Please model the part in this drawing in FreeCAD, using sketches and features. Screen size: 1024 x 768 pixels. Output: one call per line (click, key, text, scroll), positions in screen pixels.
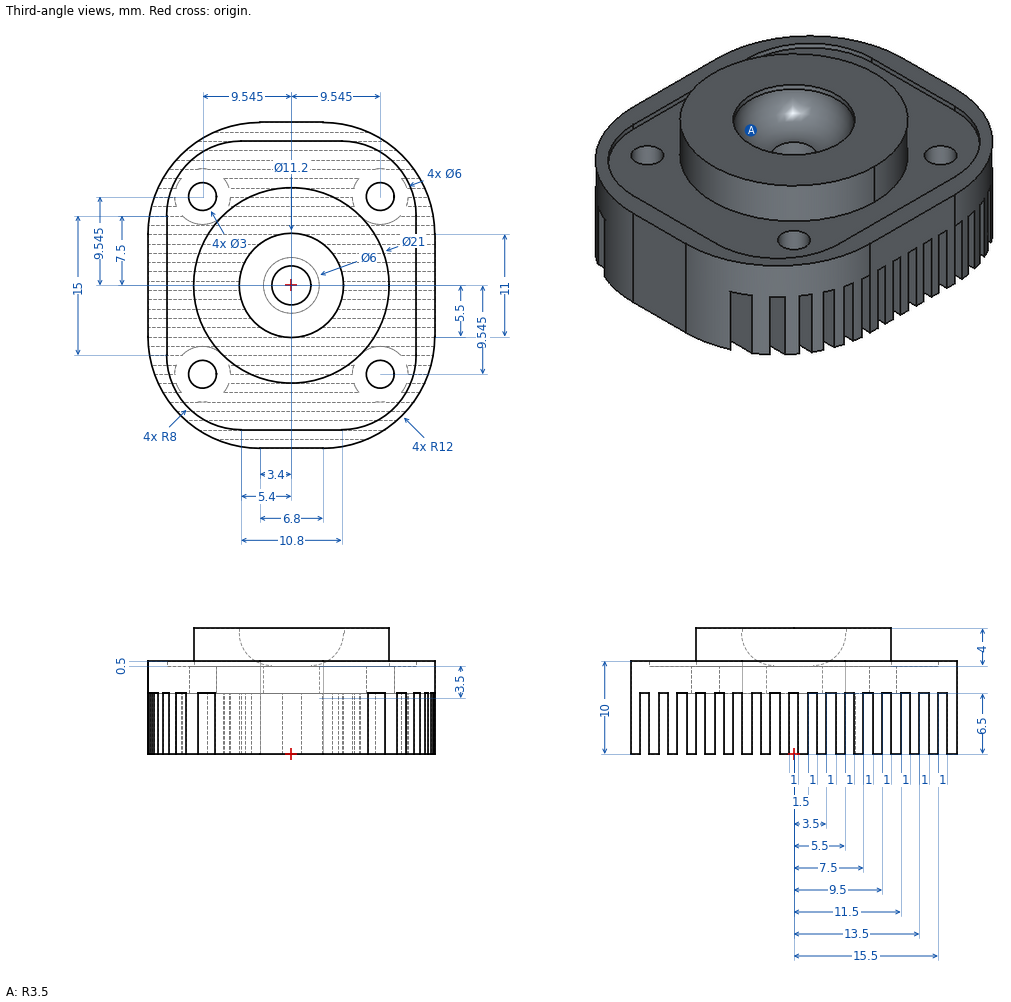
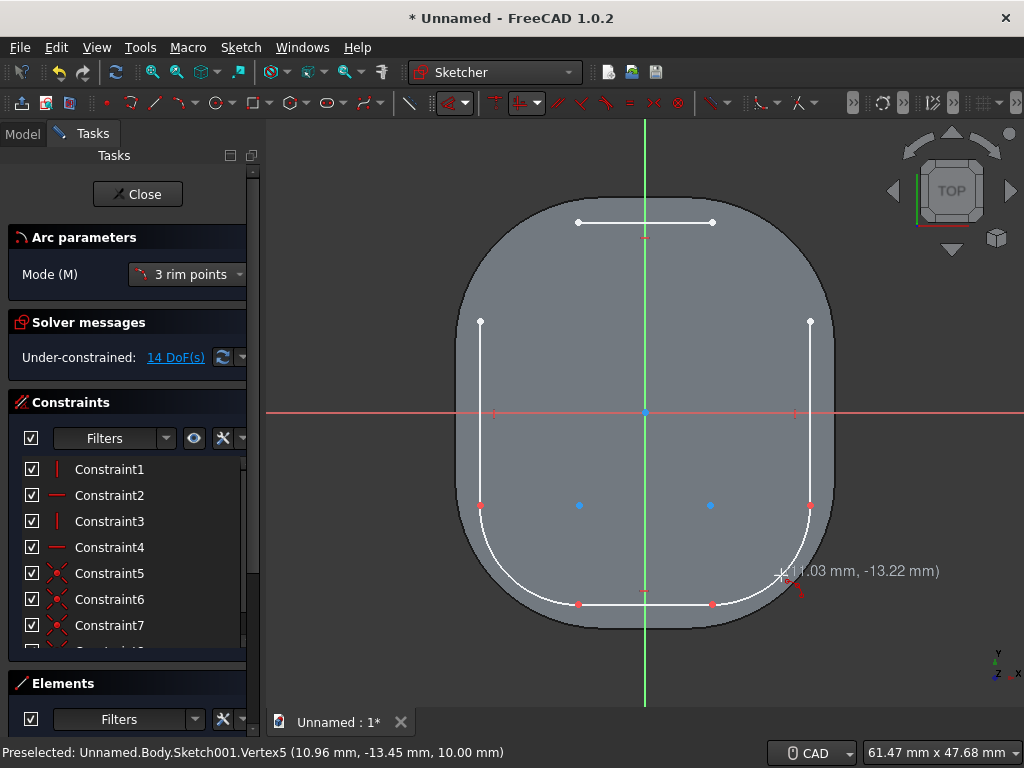
click(810, 322)
click(712, 223)
click(781, 251)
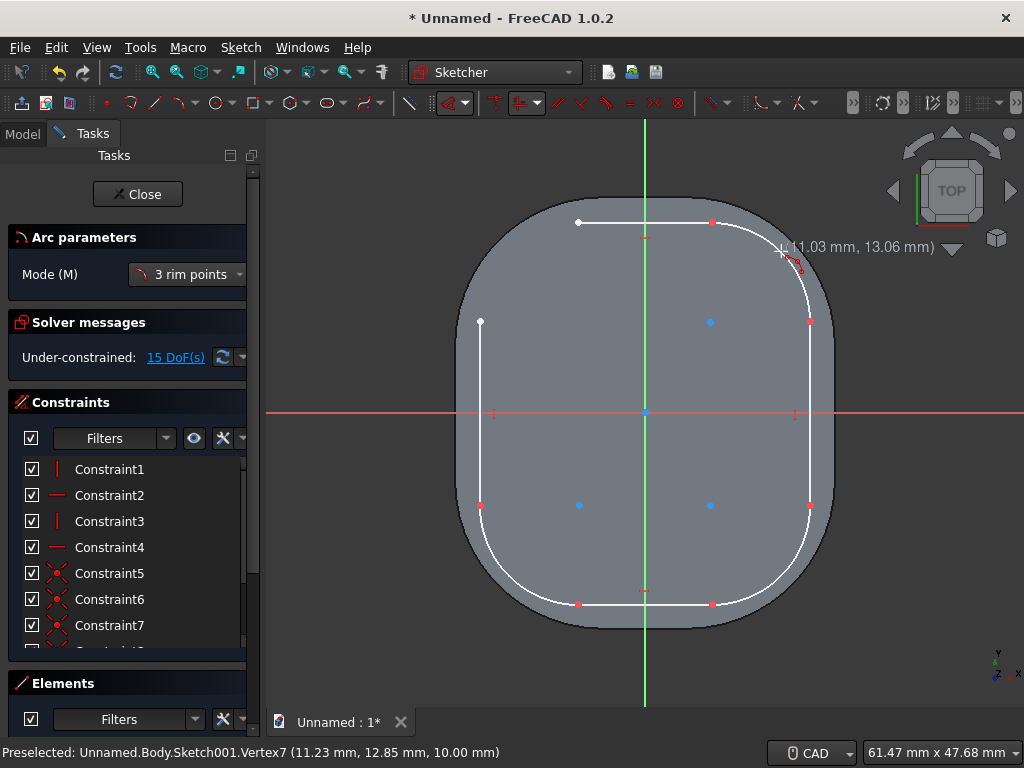
click(578, 223)
click(480, 322)
click(509, 251)
key(Escape)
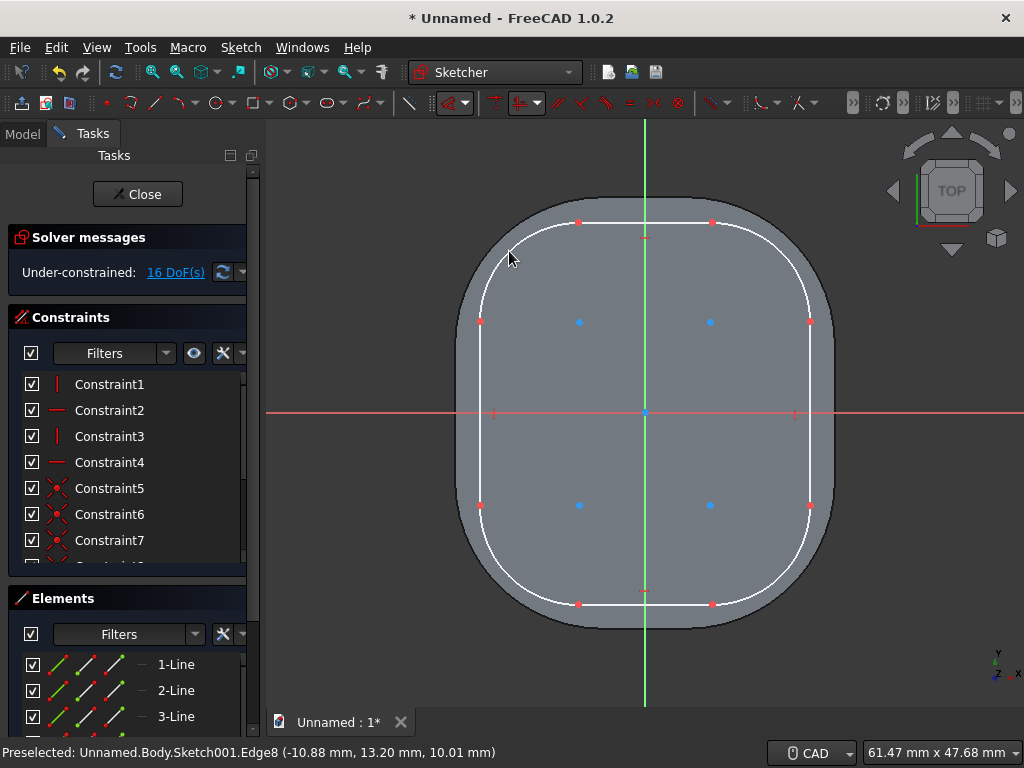
click(480, 377)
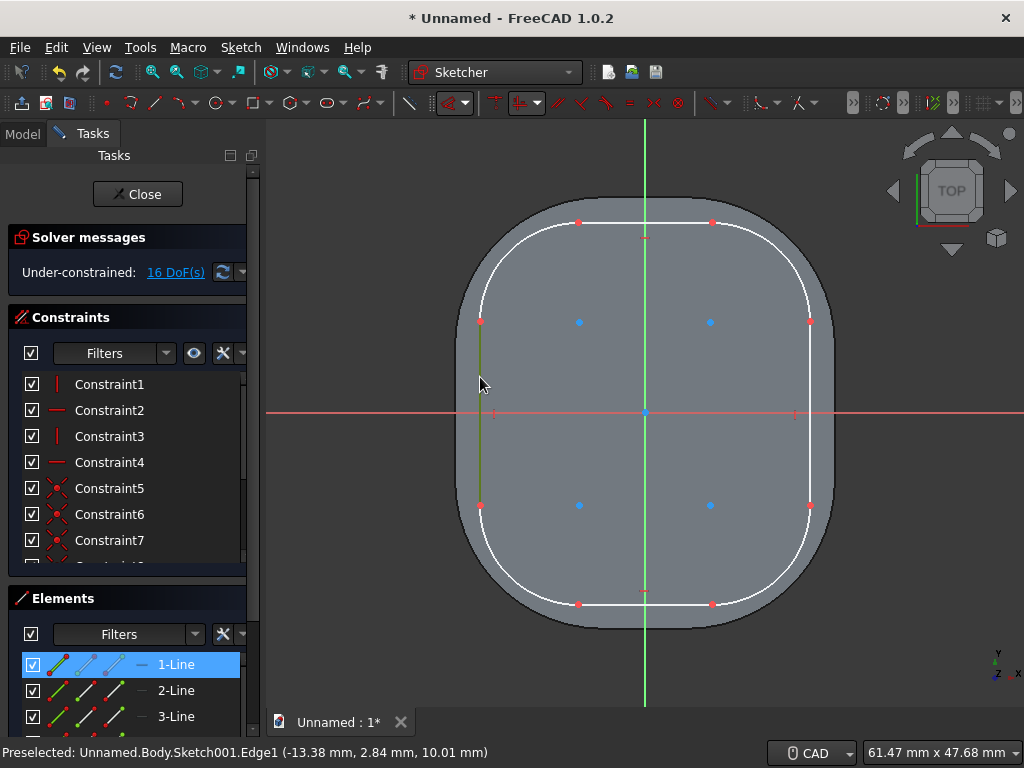
click(491, 551)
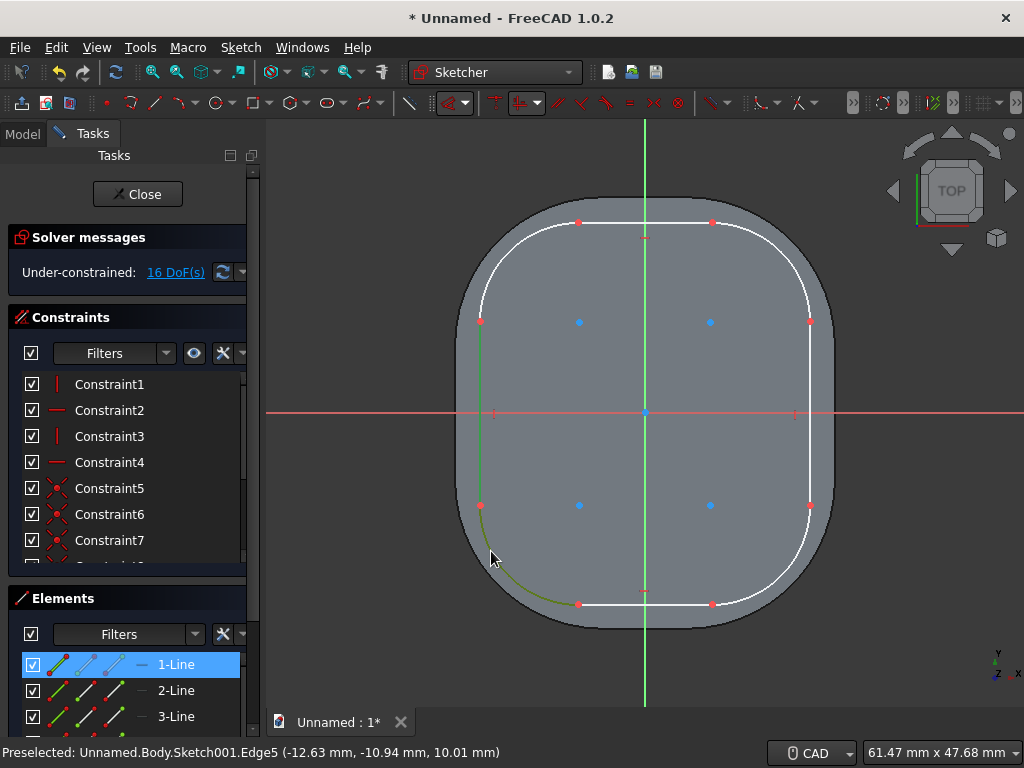
click(606, 104)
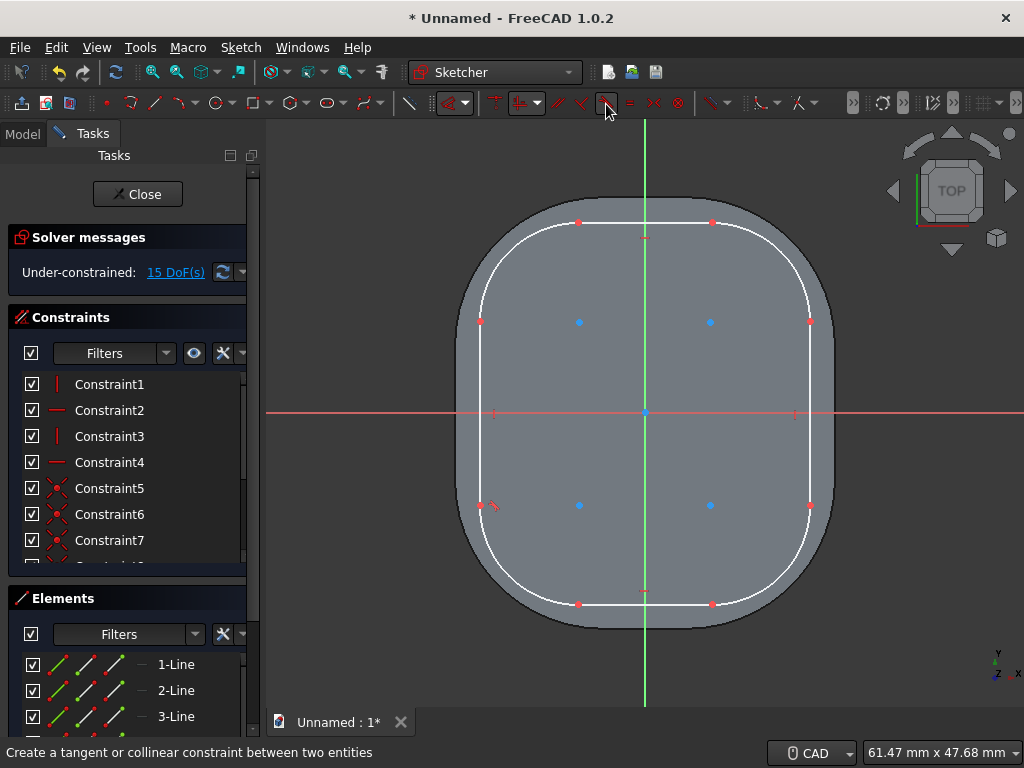
click(480, 377)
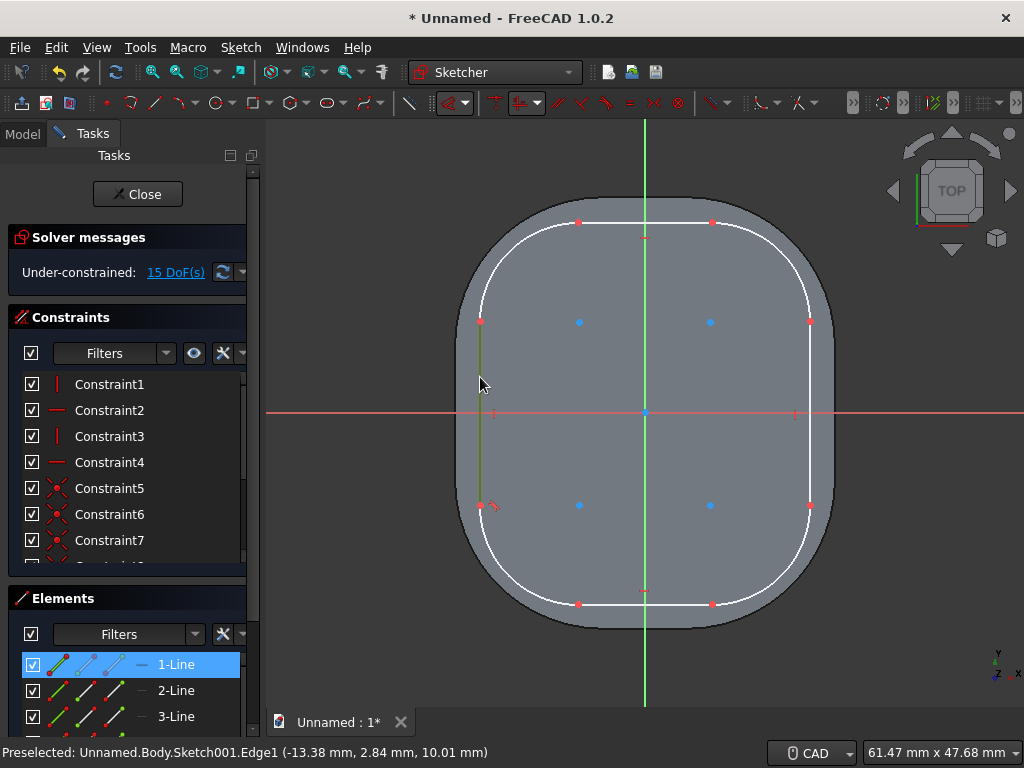
click(533, 234)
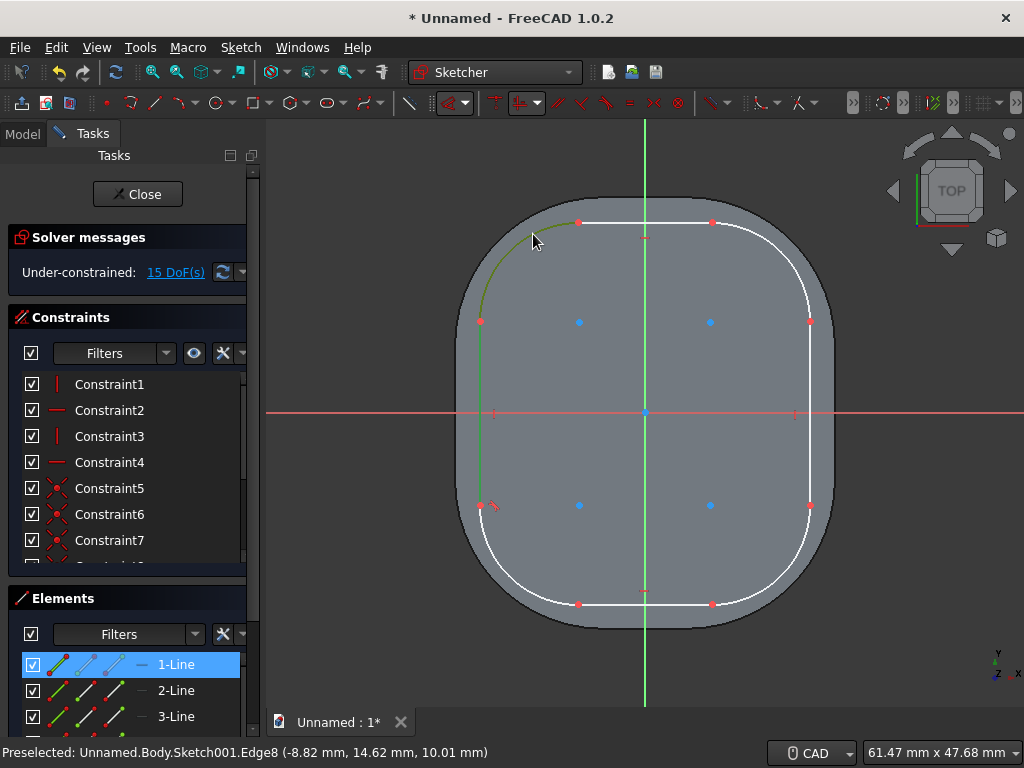
click(606, 104)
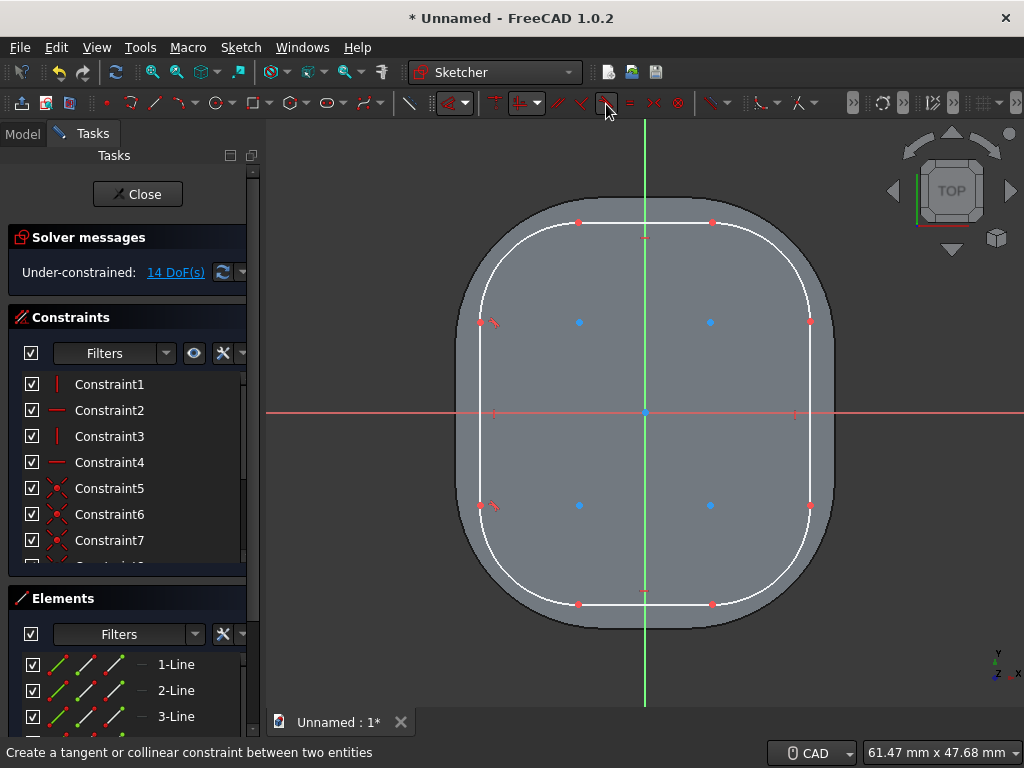
click(618, 605)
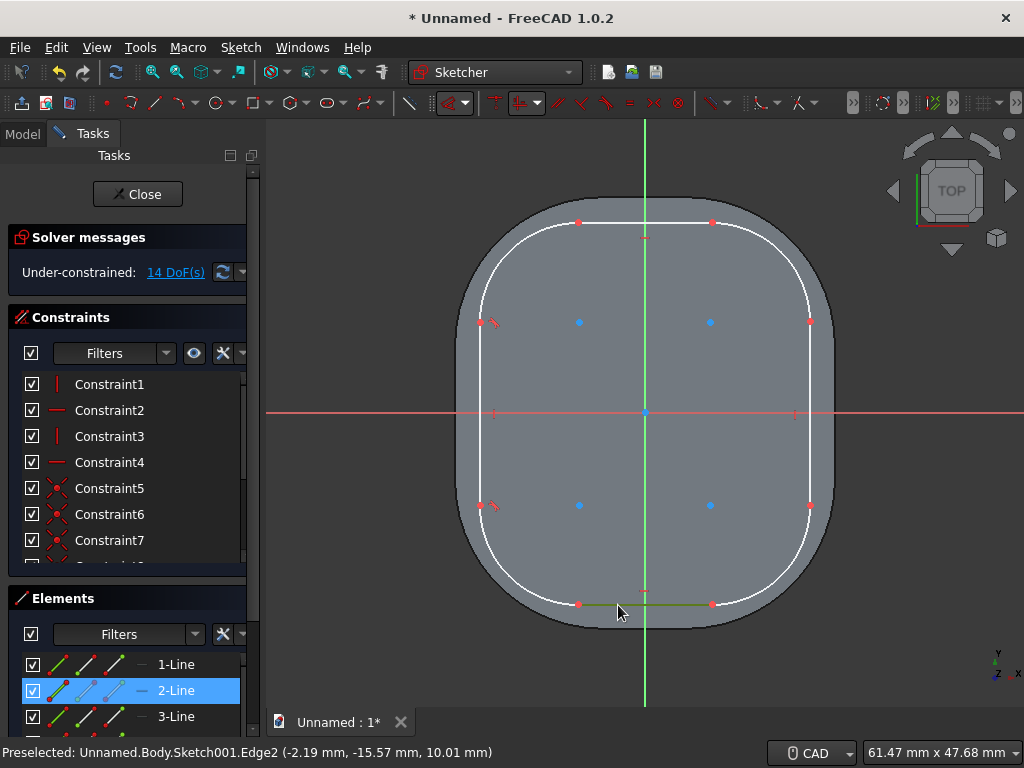
click(491, 551)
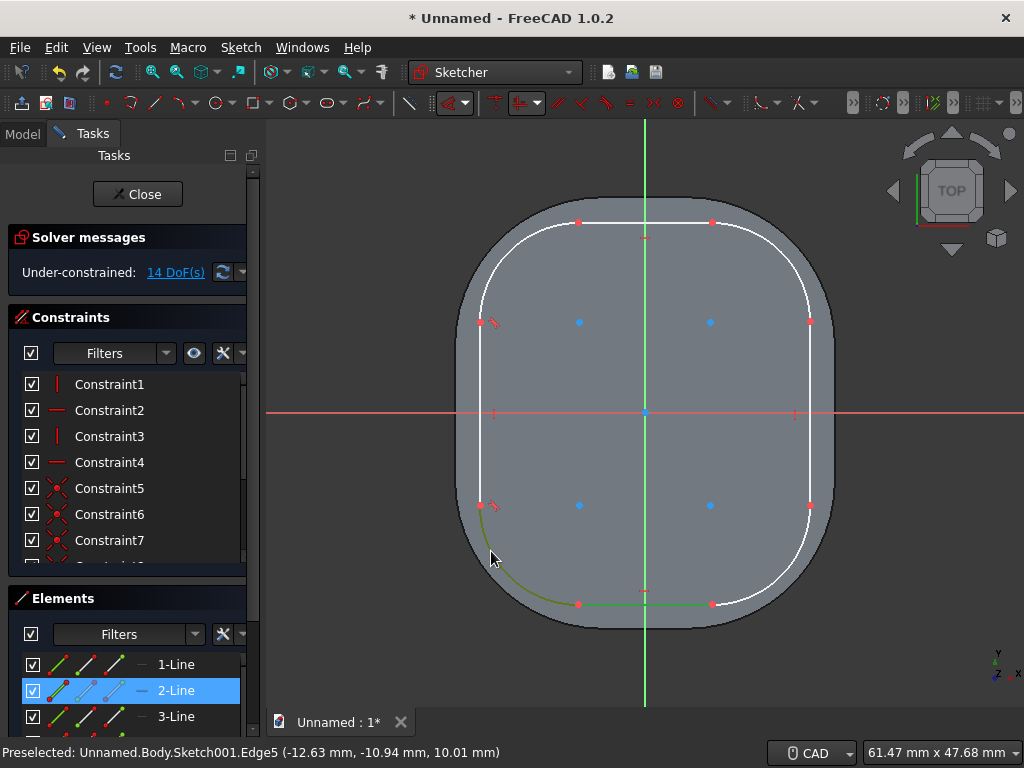
click(606, 104)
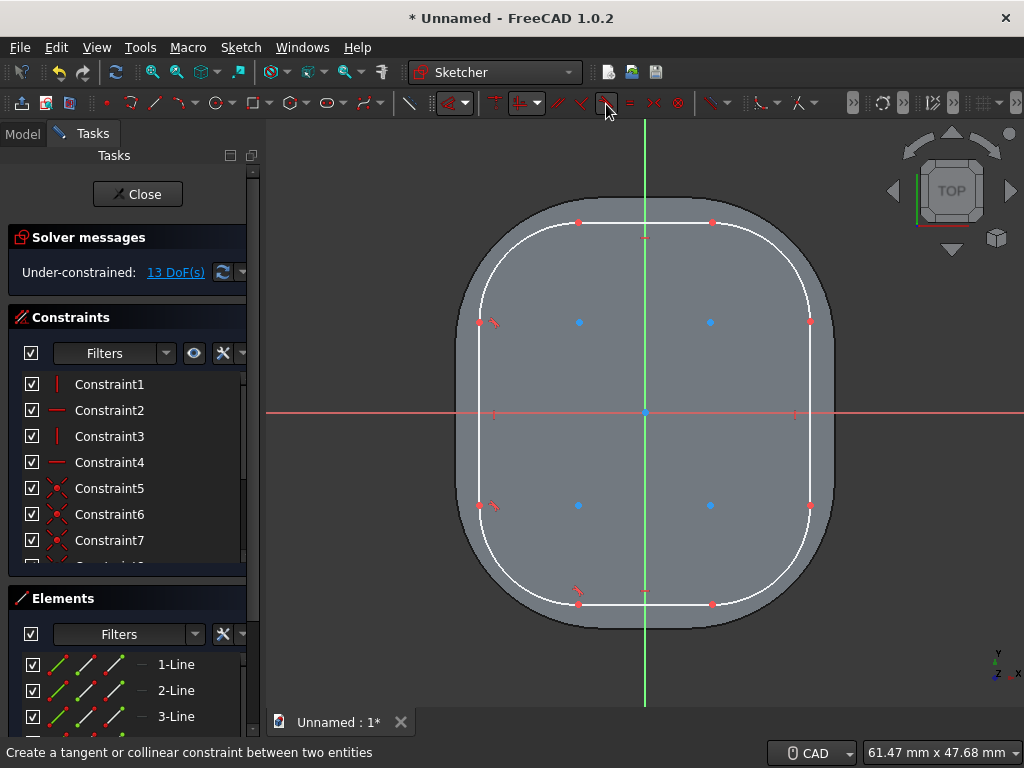
click(619, 605)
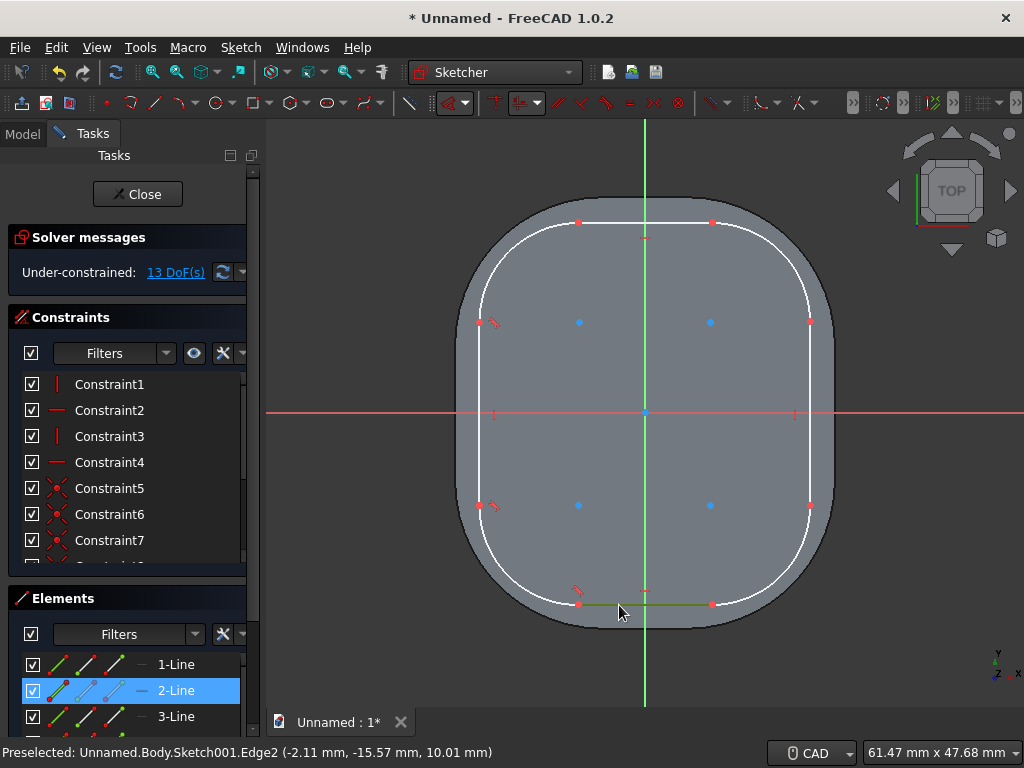
click(757, 594)